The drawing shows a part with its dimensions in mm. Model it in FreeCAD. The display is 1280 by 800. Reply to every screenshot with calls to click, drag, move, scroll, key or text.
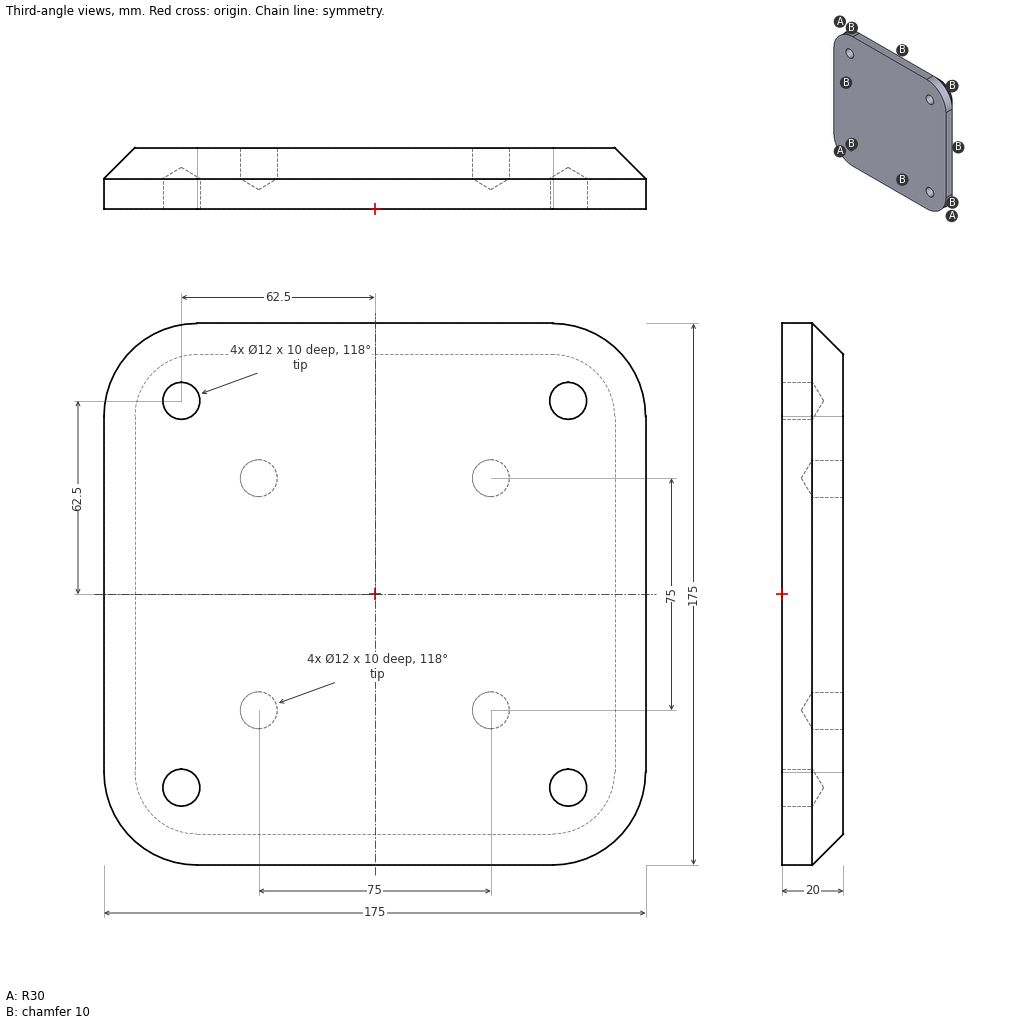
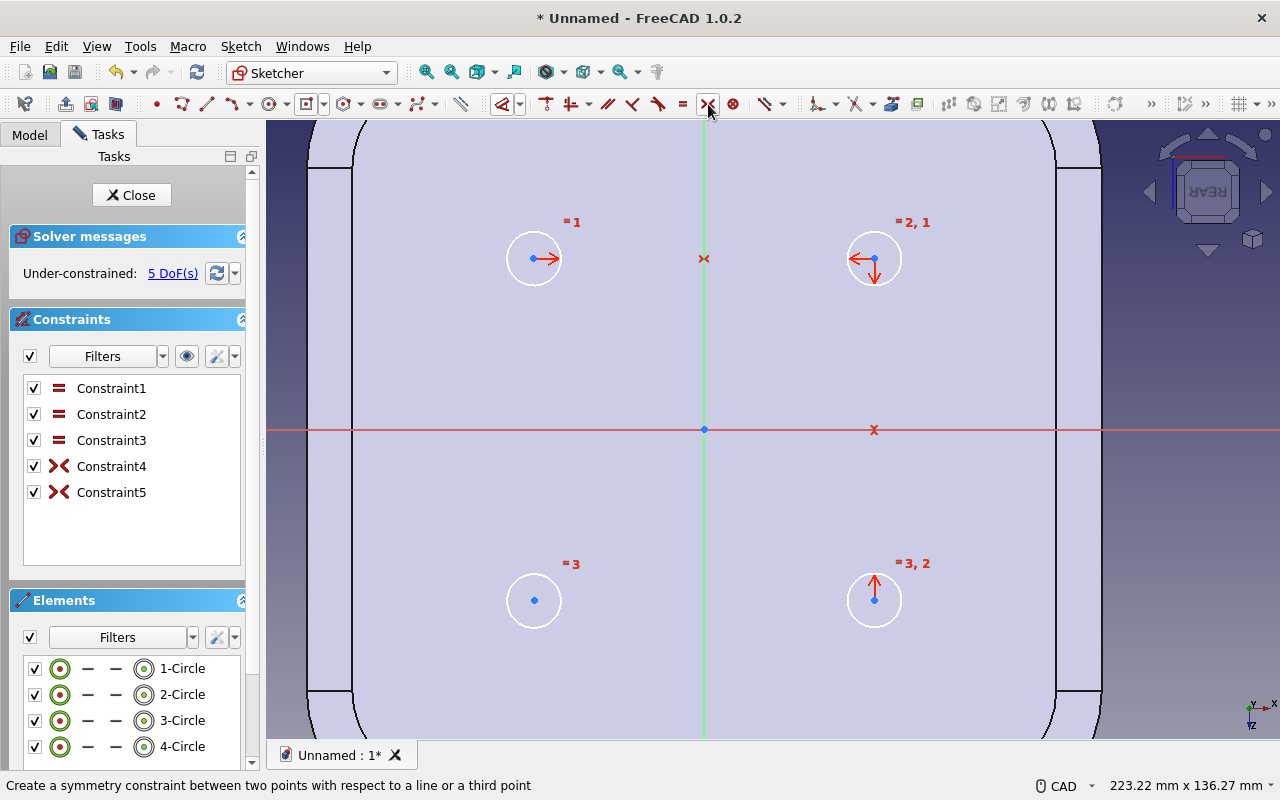
click(534, 259)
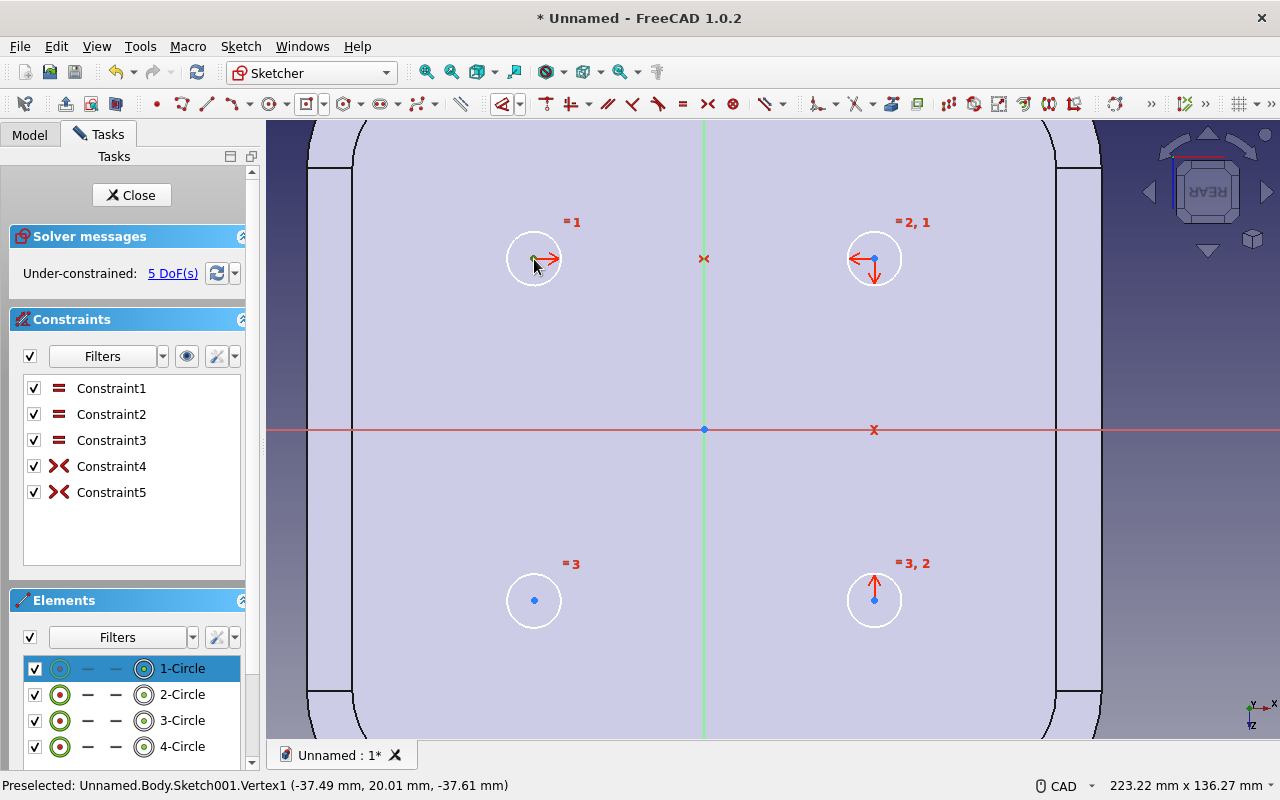
click(534, 601)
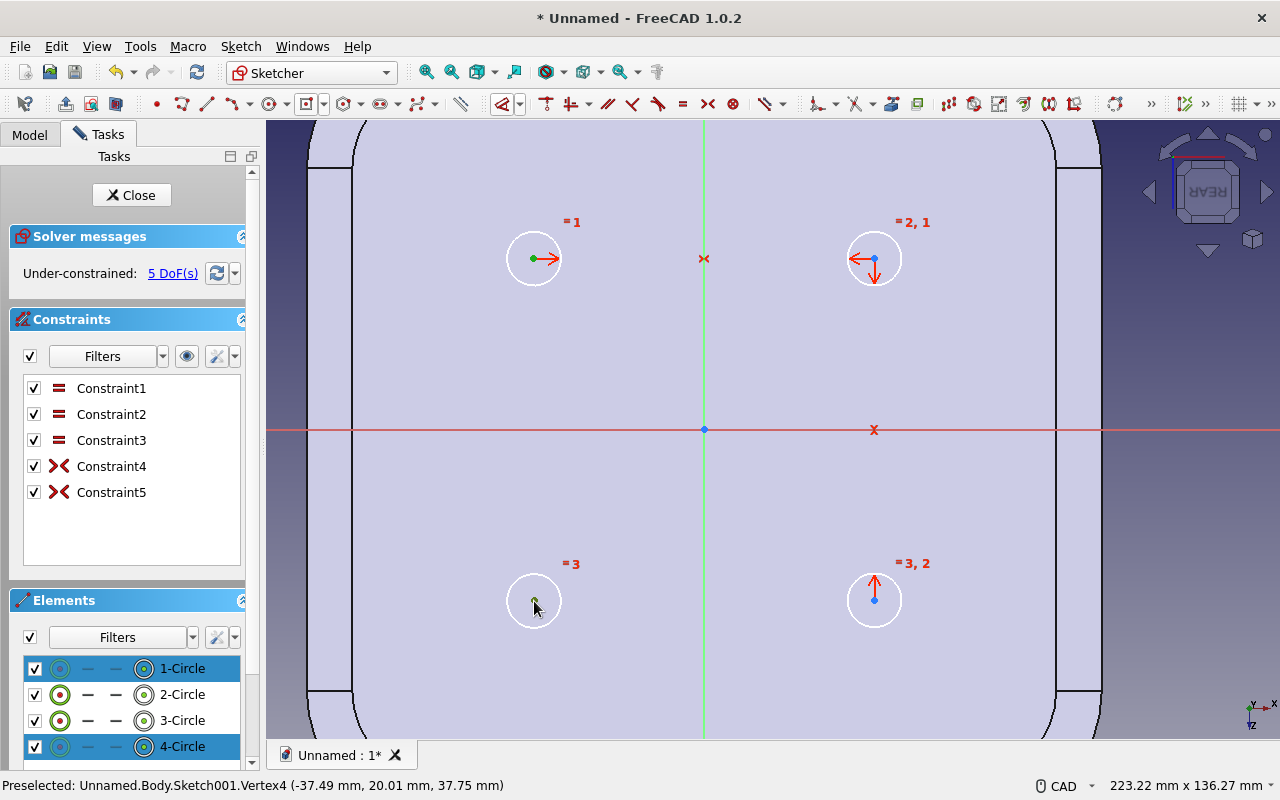
click(353, 429)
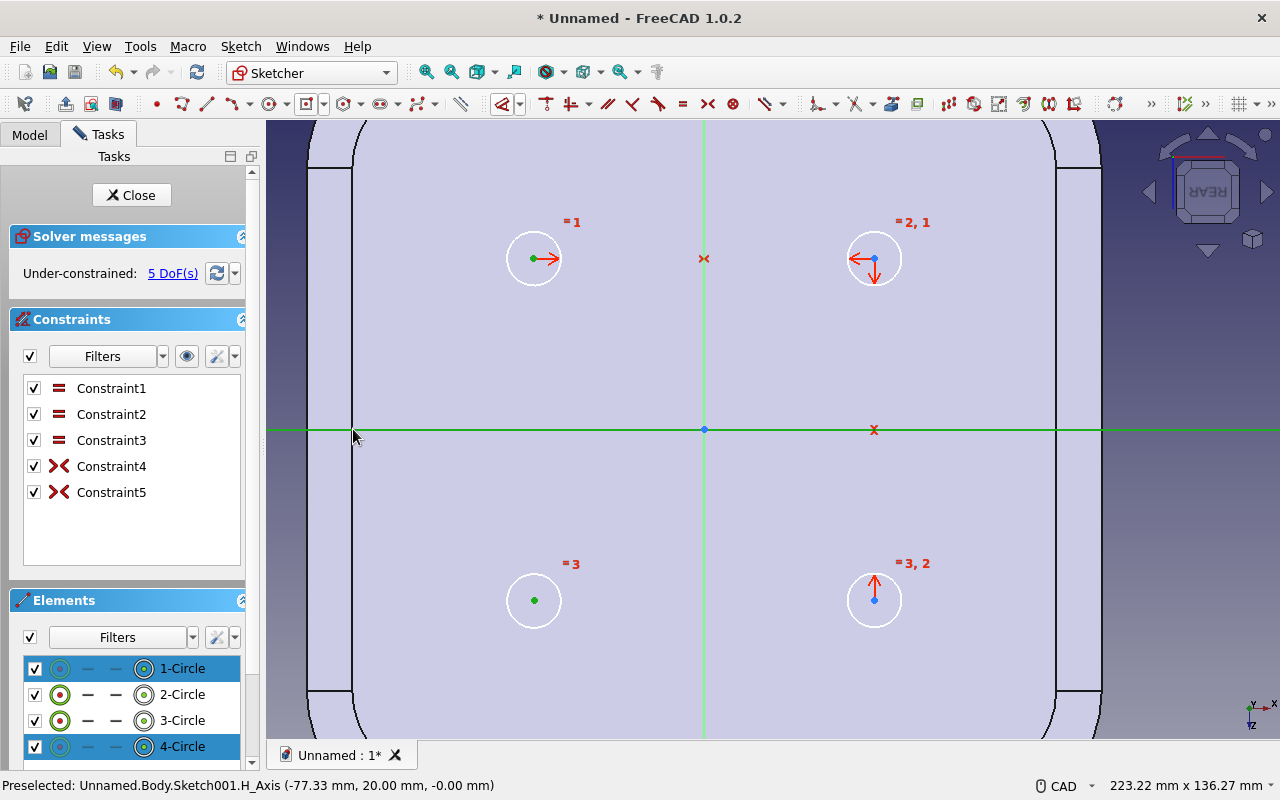
click(708, 104)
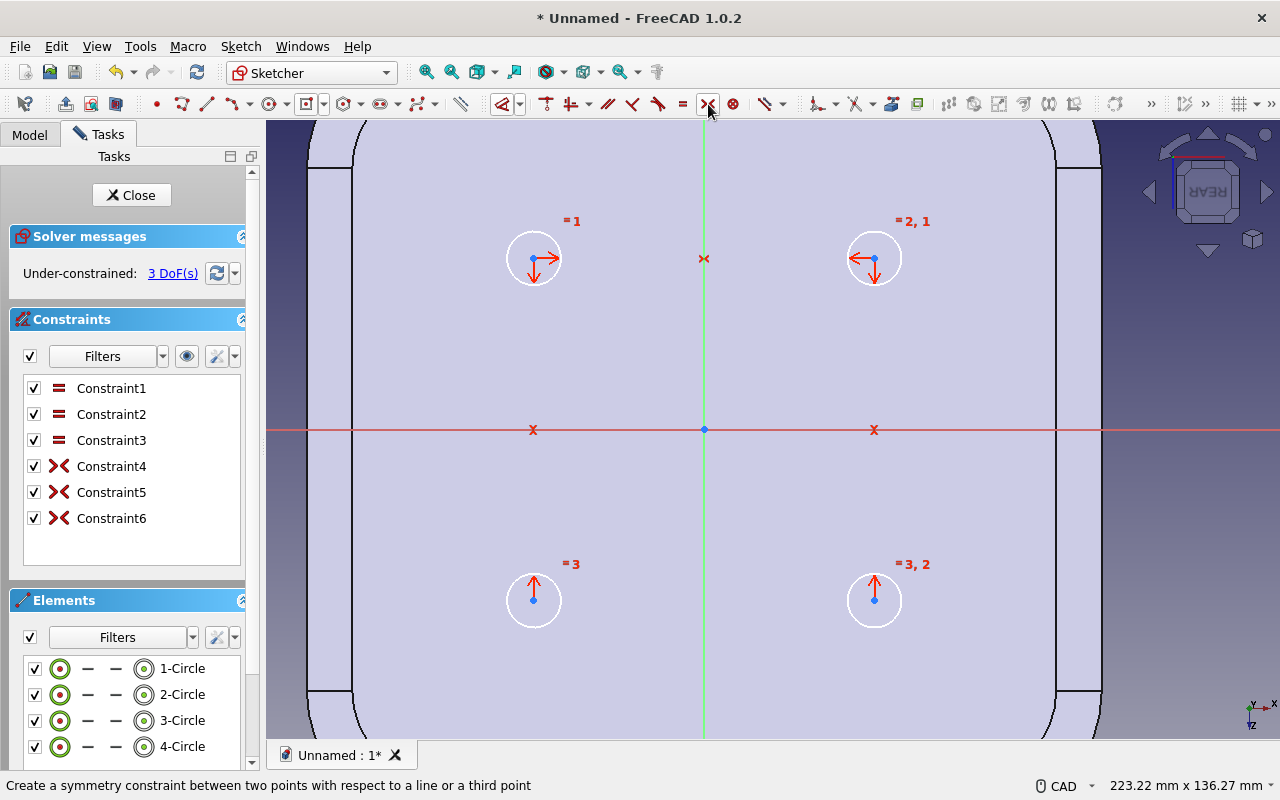
click(553, 239)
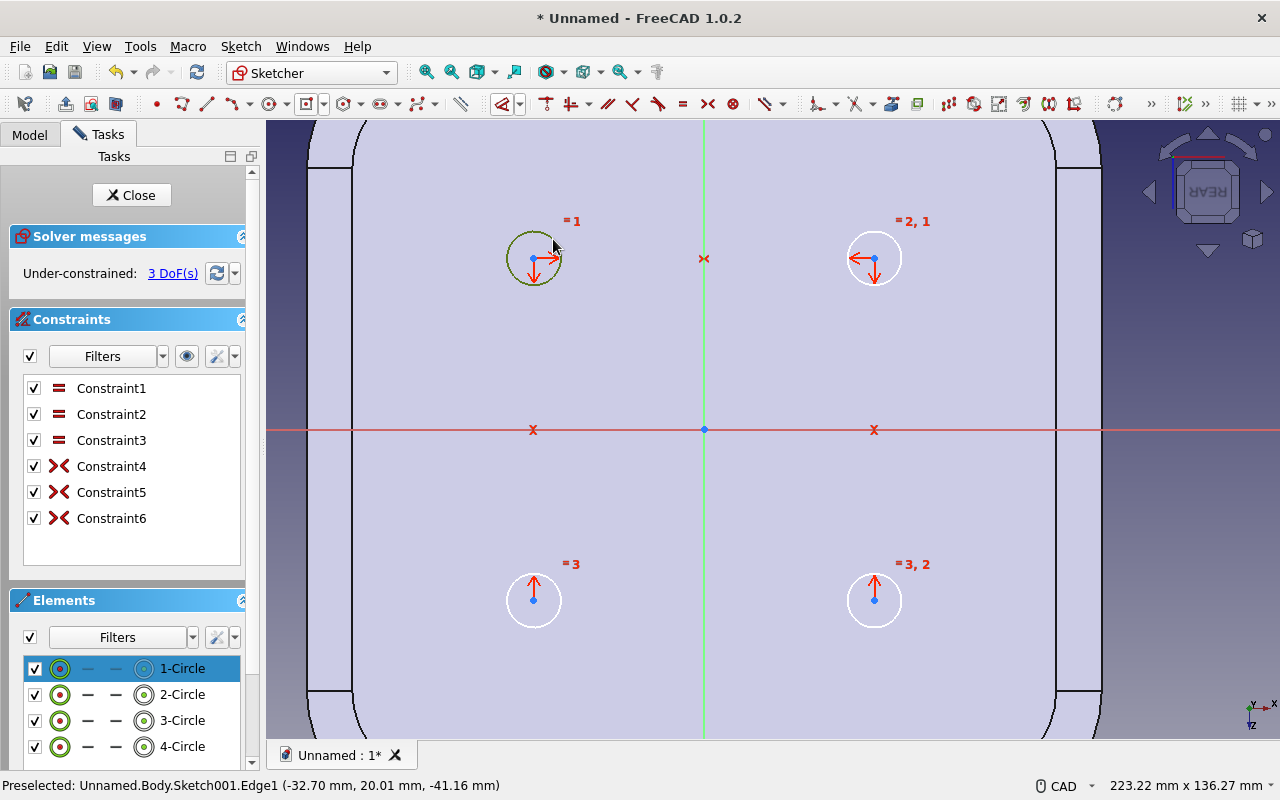
key(k)
key(o)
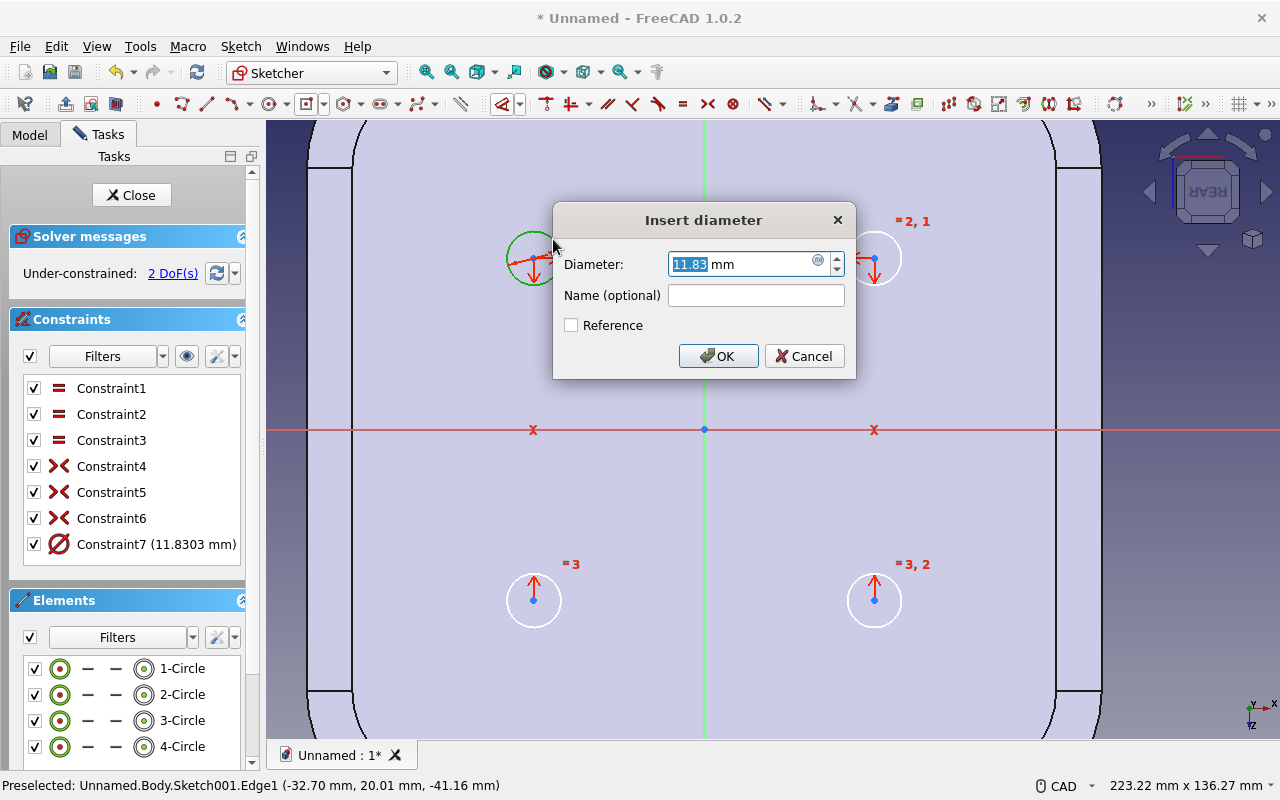
text(12)
key(Return)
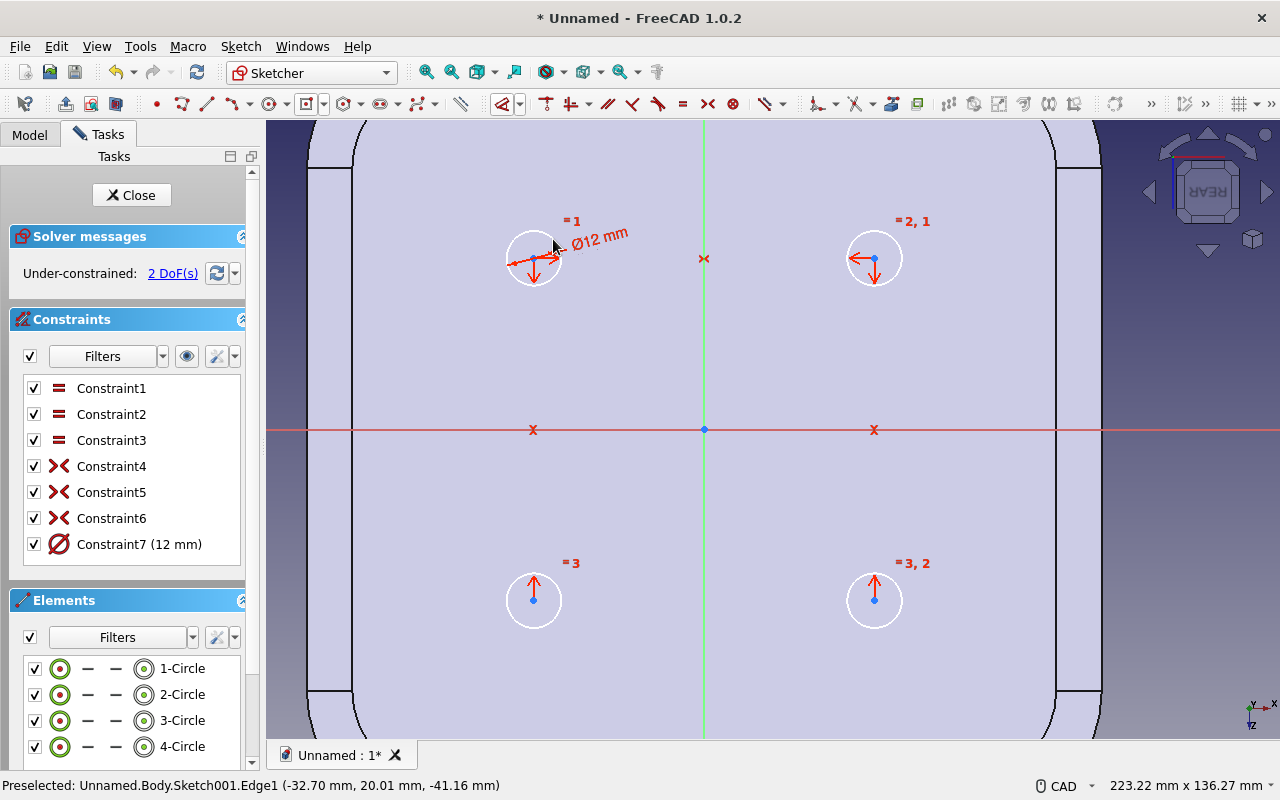
click(534, 258)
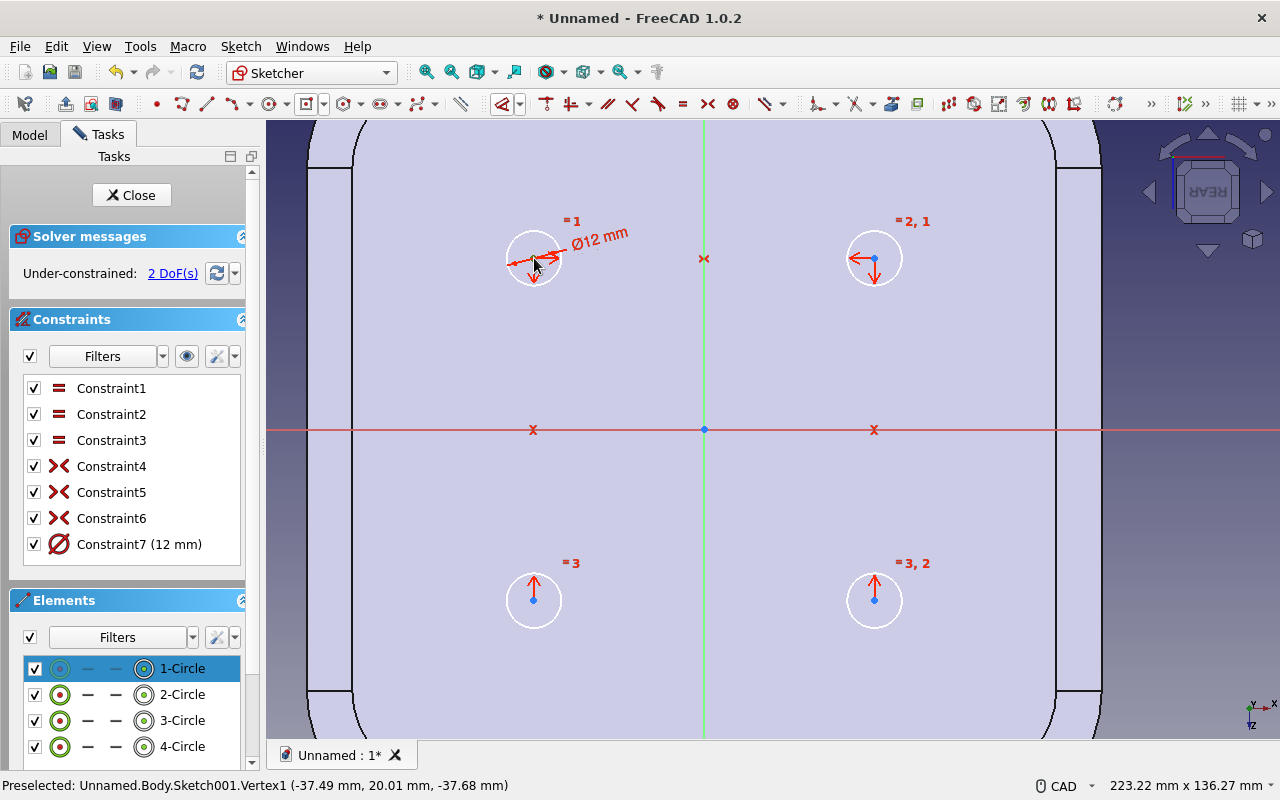
click(875, 258)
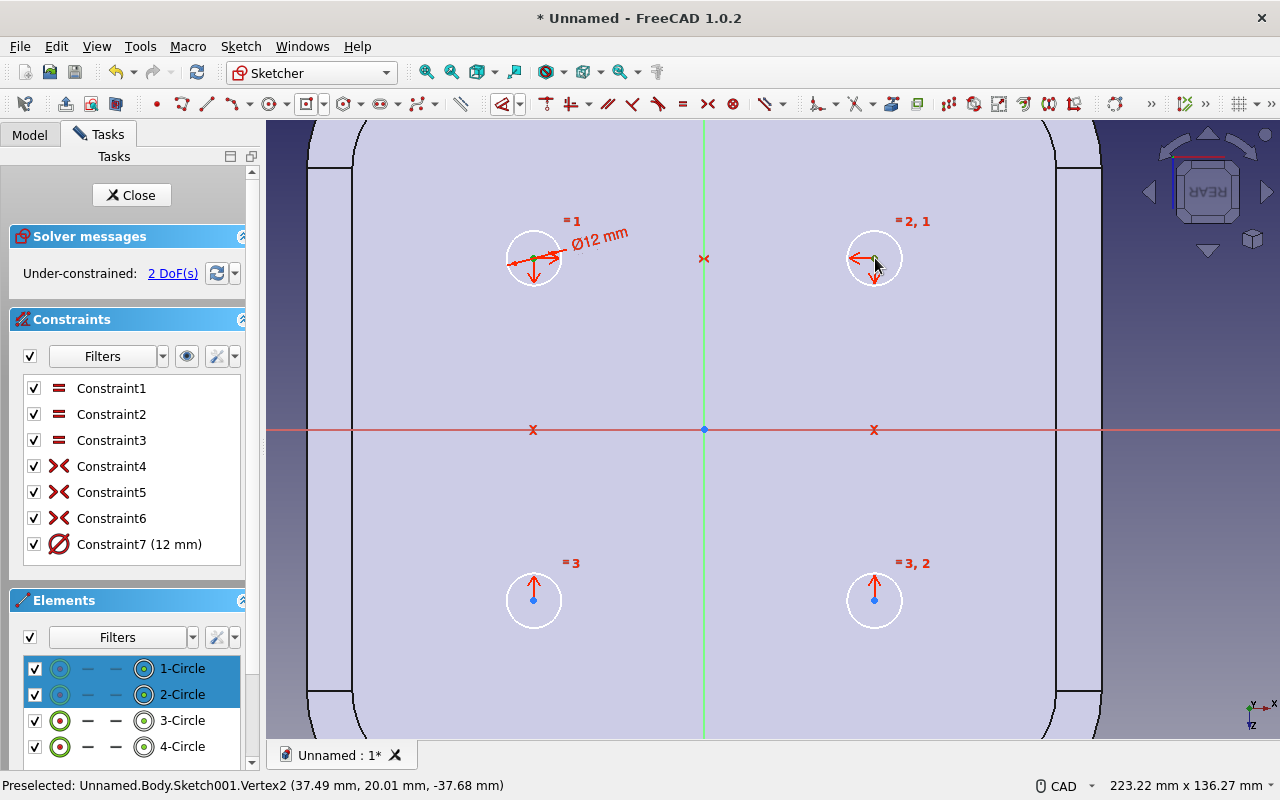
key(l)